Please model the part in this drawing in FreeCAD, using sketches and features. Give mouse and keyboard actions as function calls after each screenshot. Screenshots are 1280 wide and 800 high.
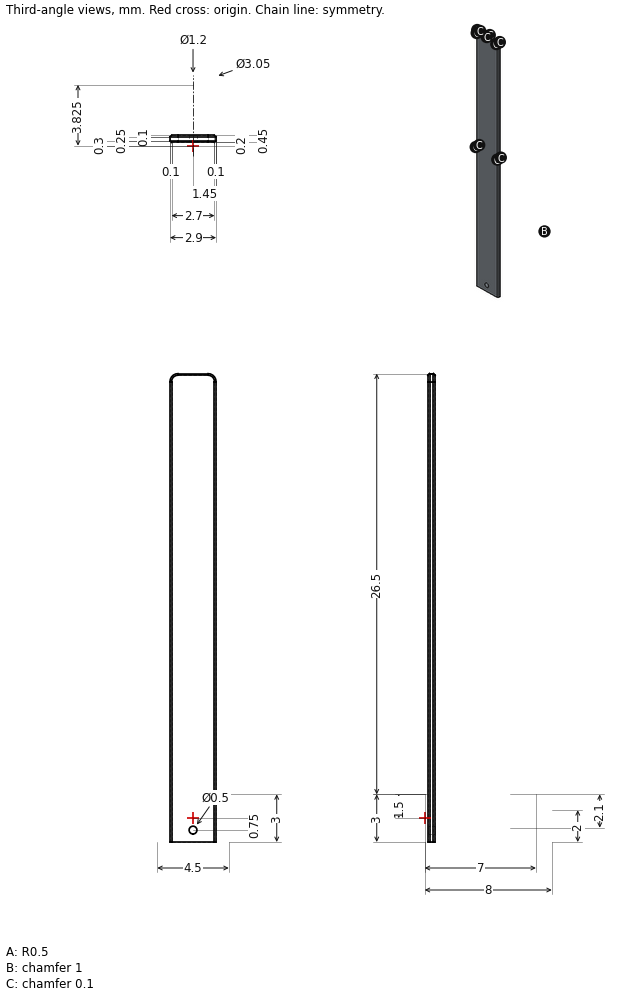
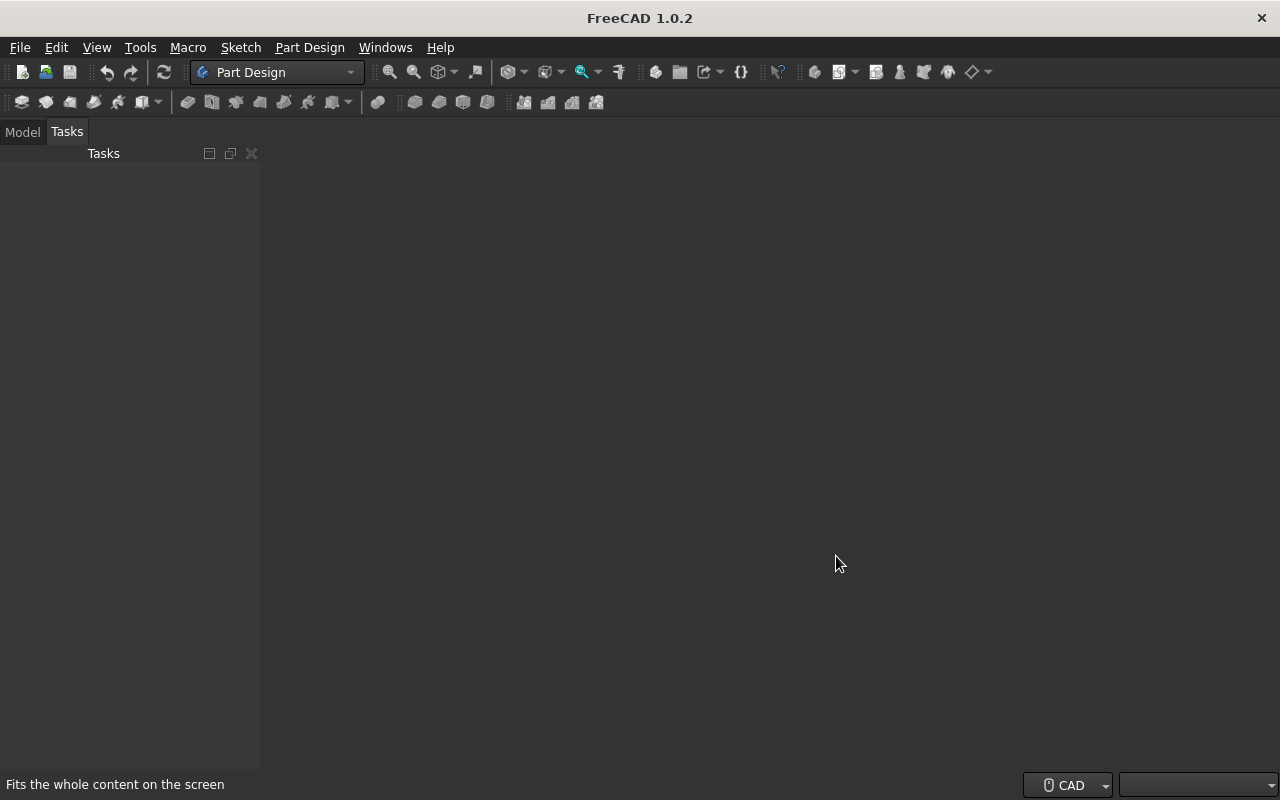
key(ctrl+n)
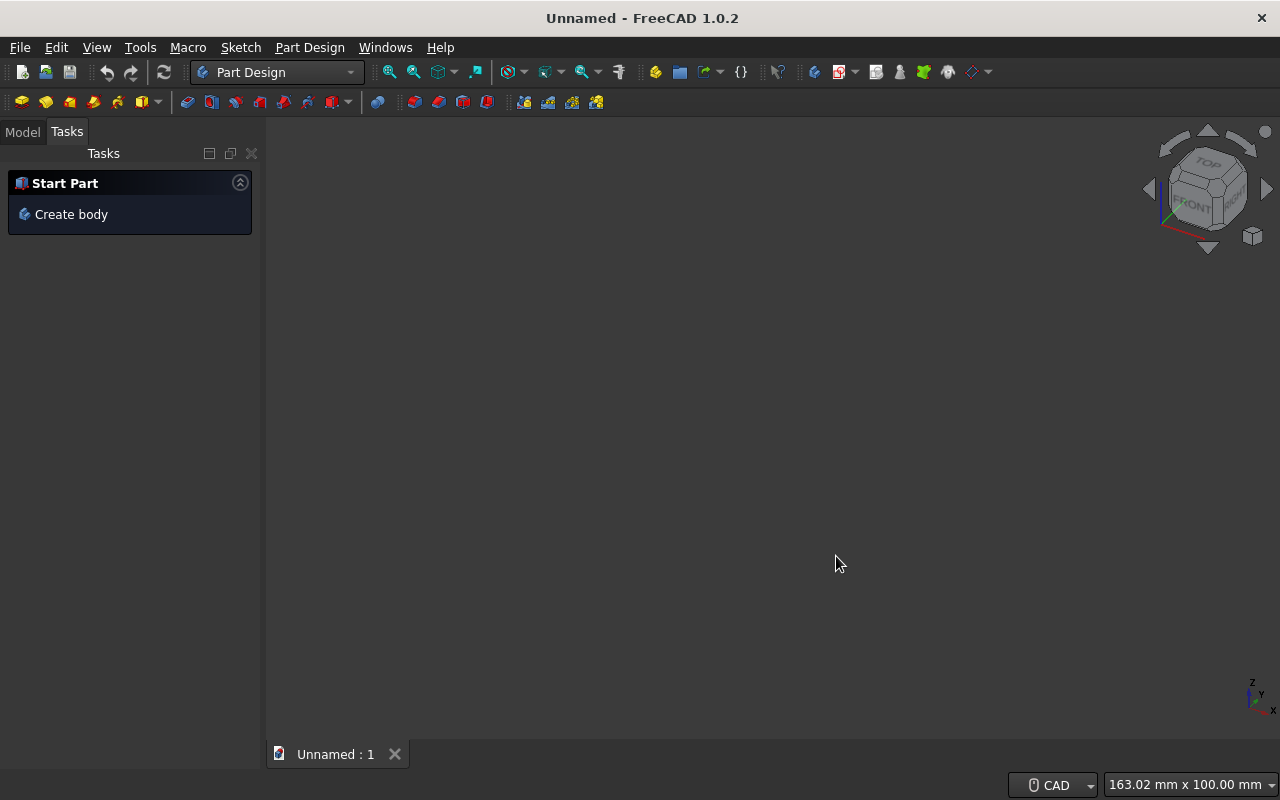
click(840, 72)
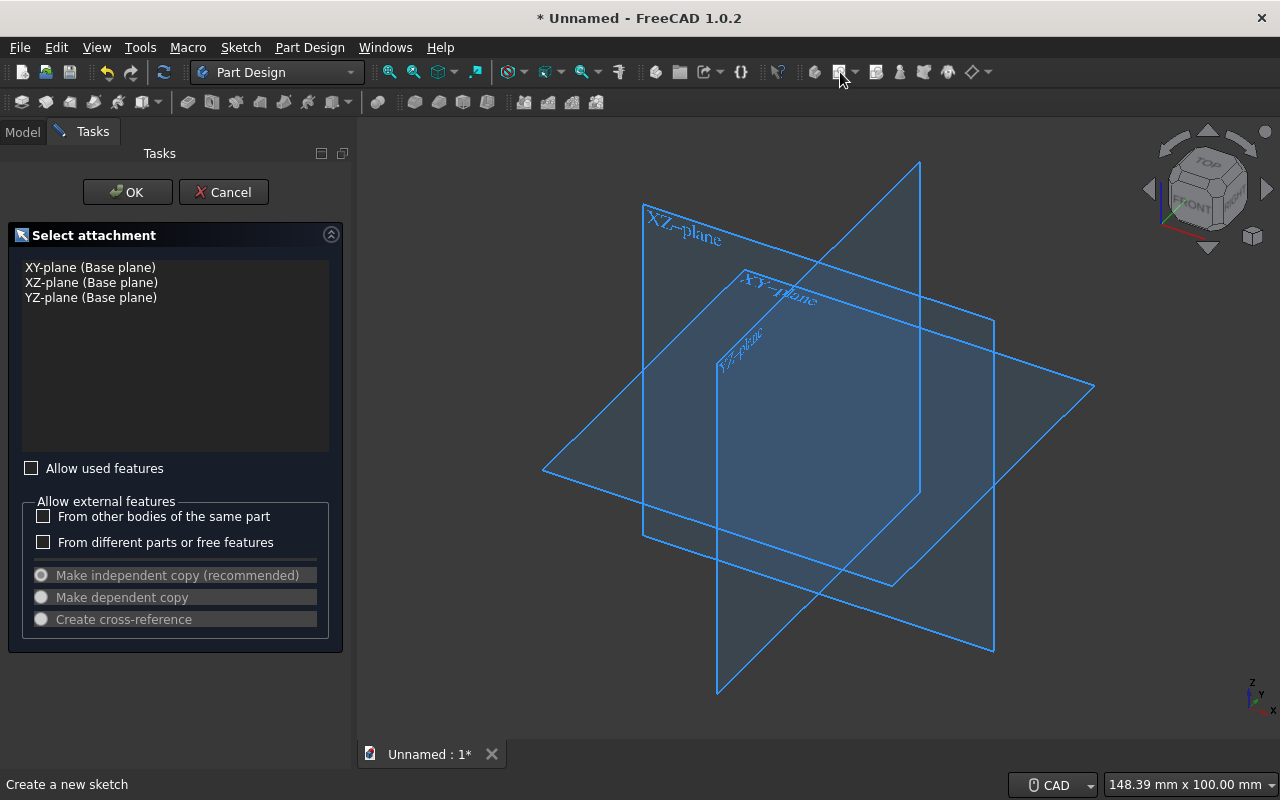
click(82, 282)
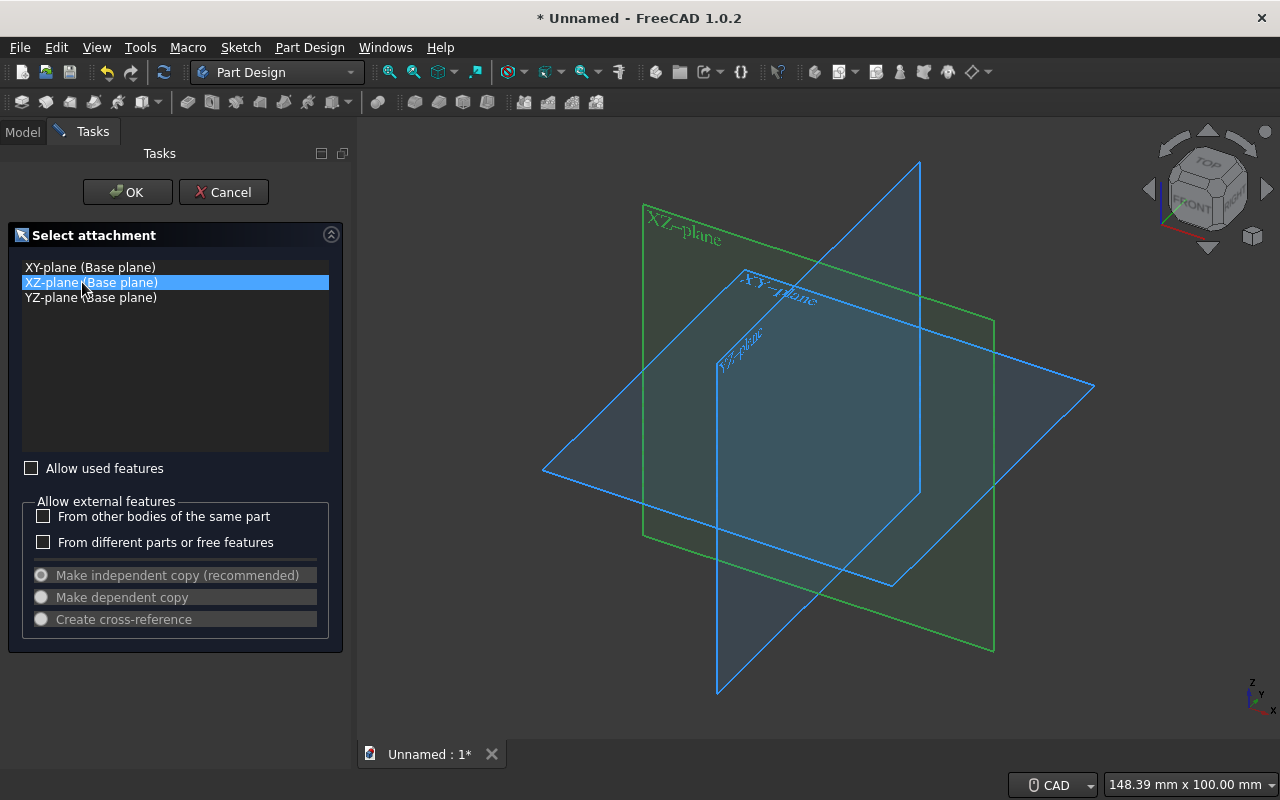
click(128, 192)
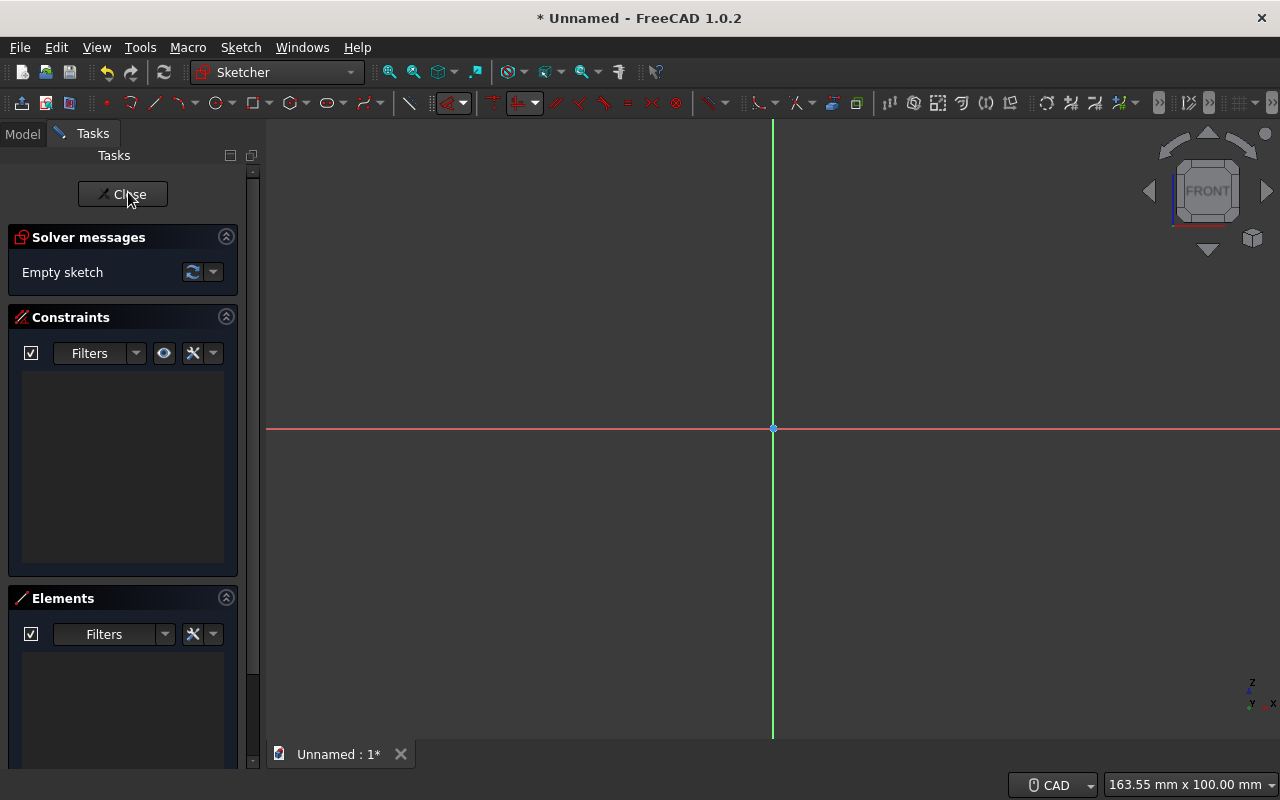
scroll(777, 429, up, 15)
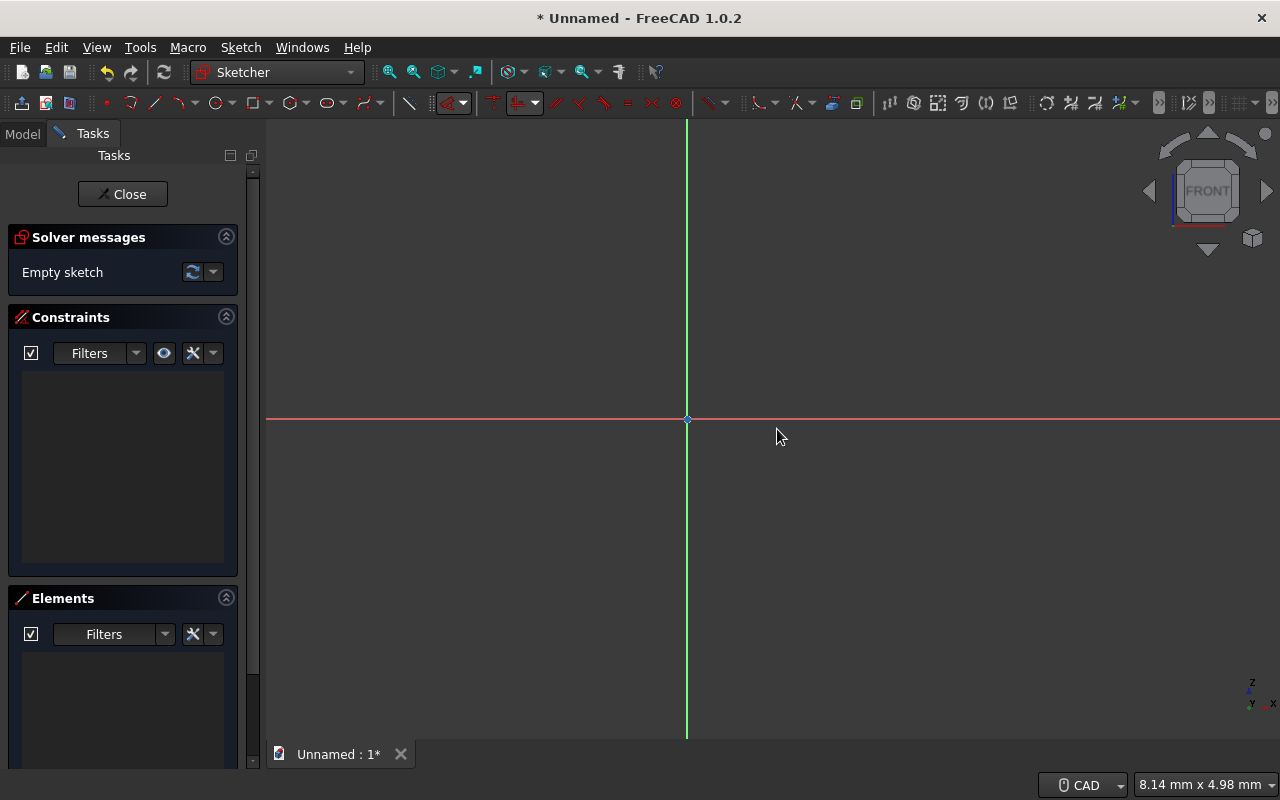
click(272, 104)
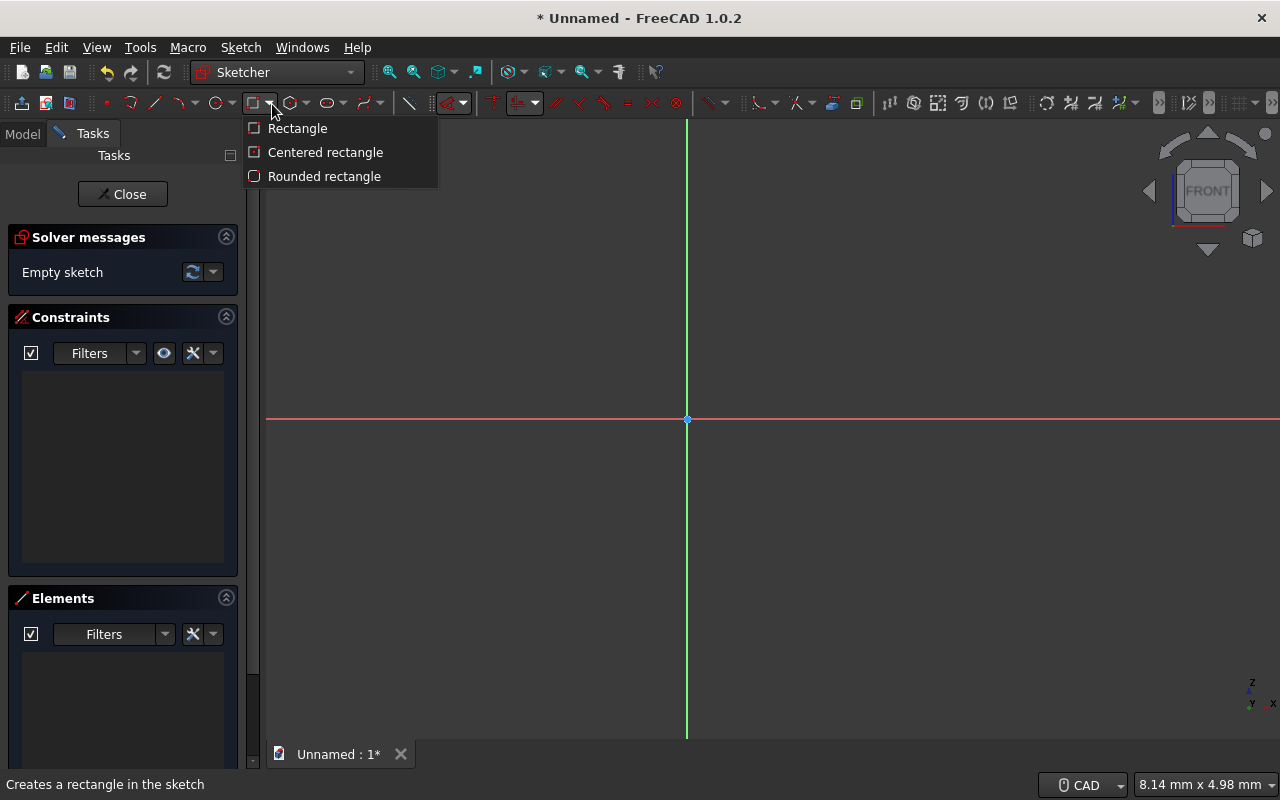
click(340, 152)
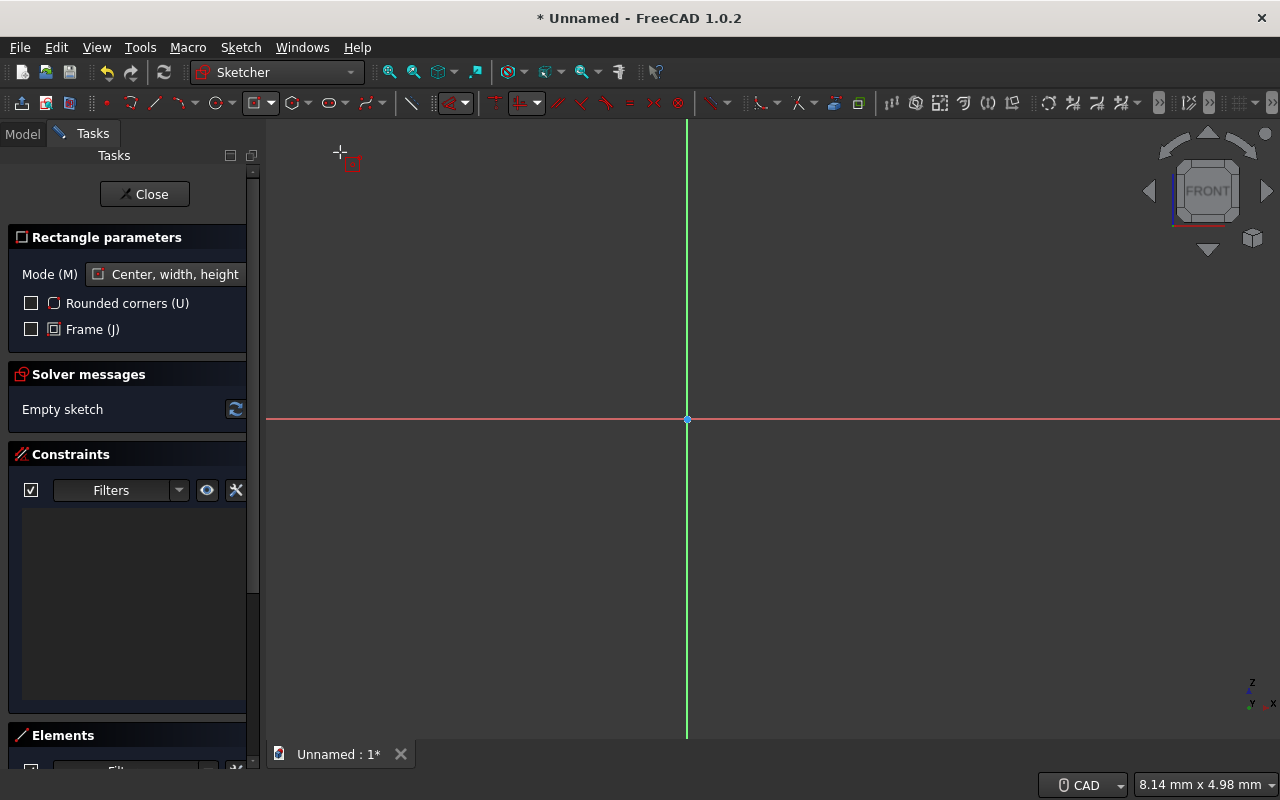
click(687, 419)
click(967, 233)
key(Escape)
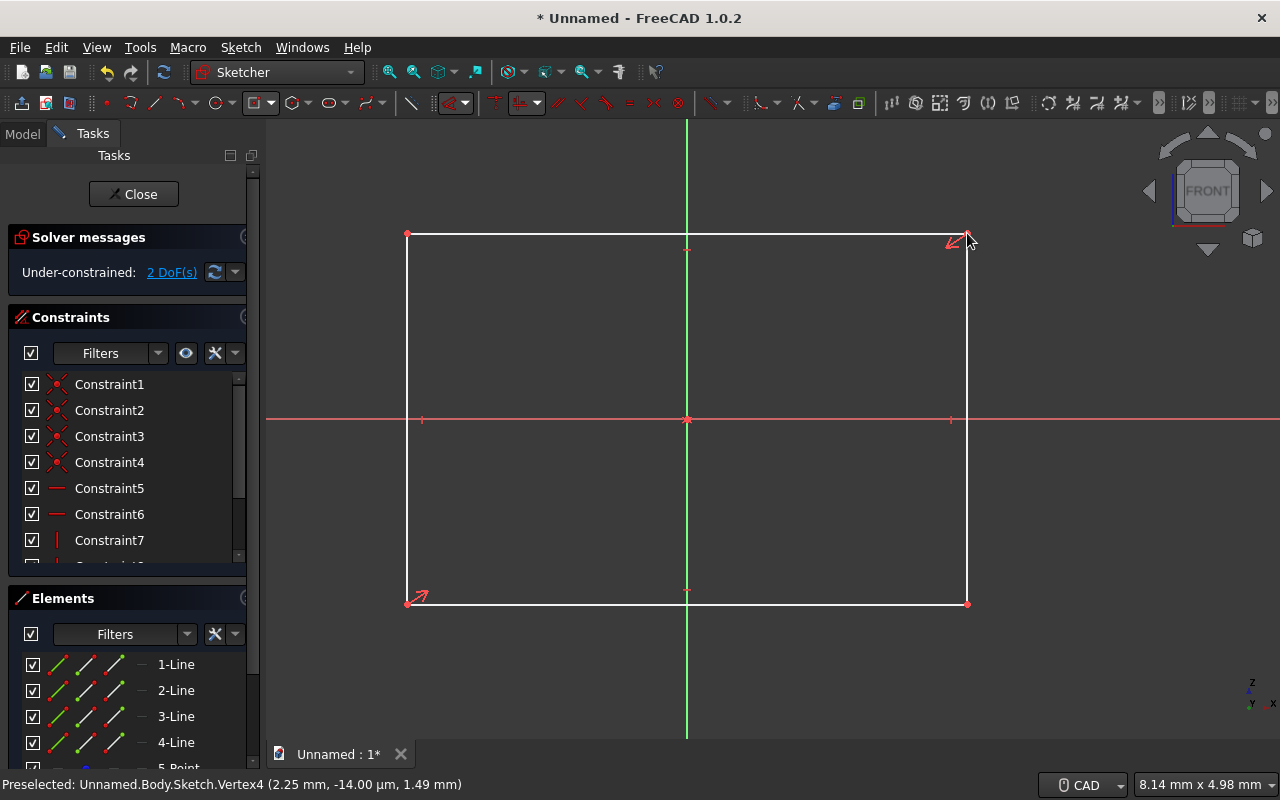
key(d)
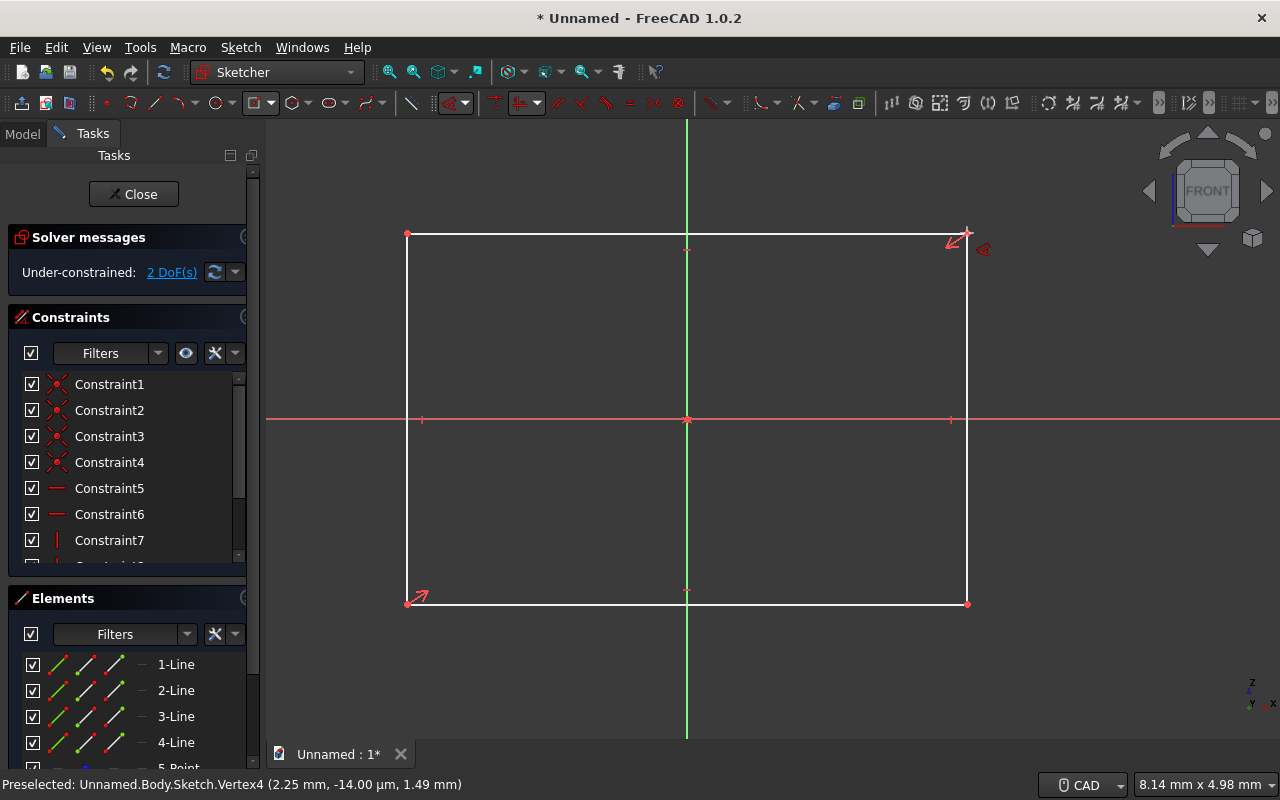
click(967, 494)
click(1001, 334)